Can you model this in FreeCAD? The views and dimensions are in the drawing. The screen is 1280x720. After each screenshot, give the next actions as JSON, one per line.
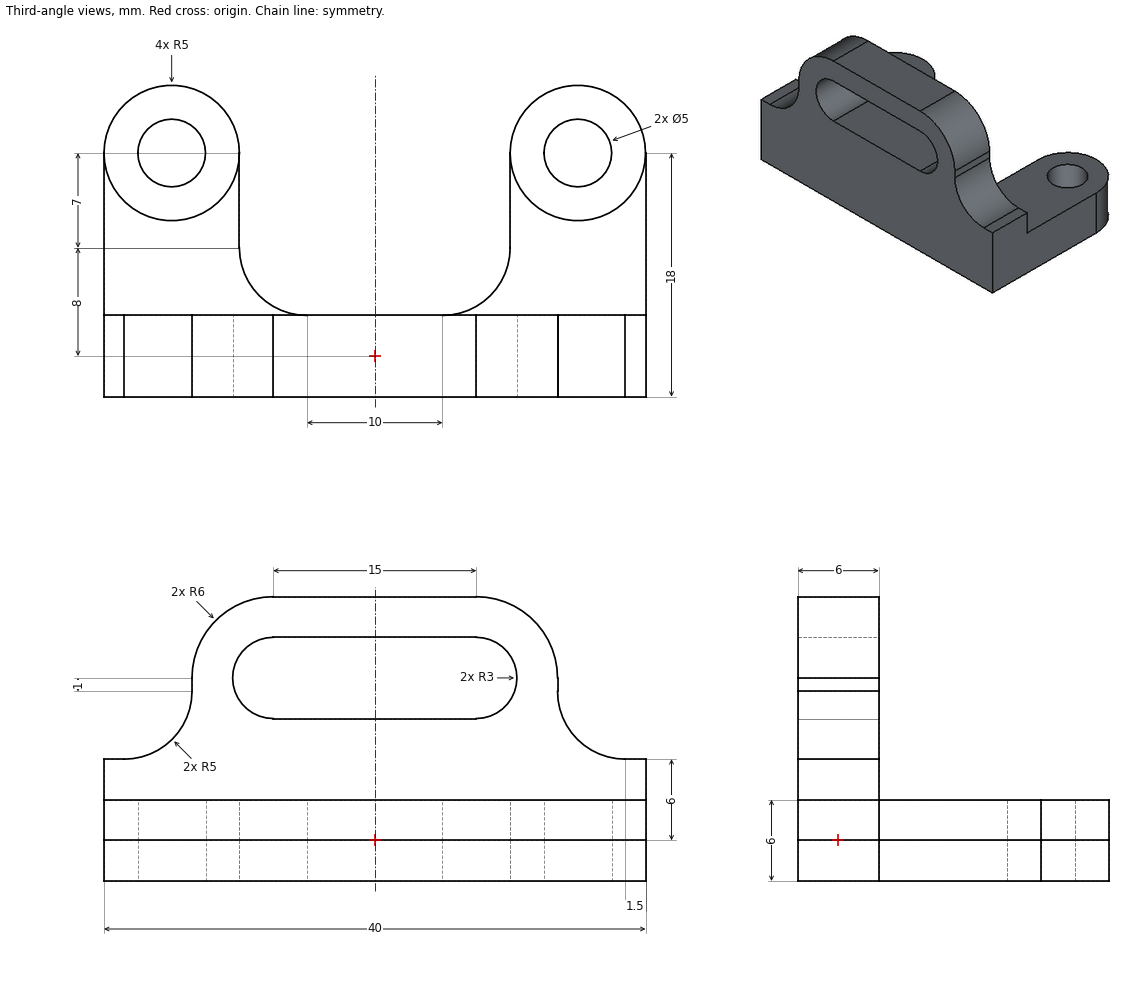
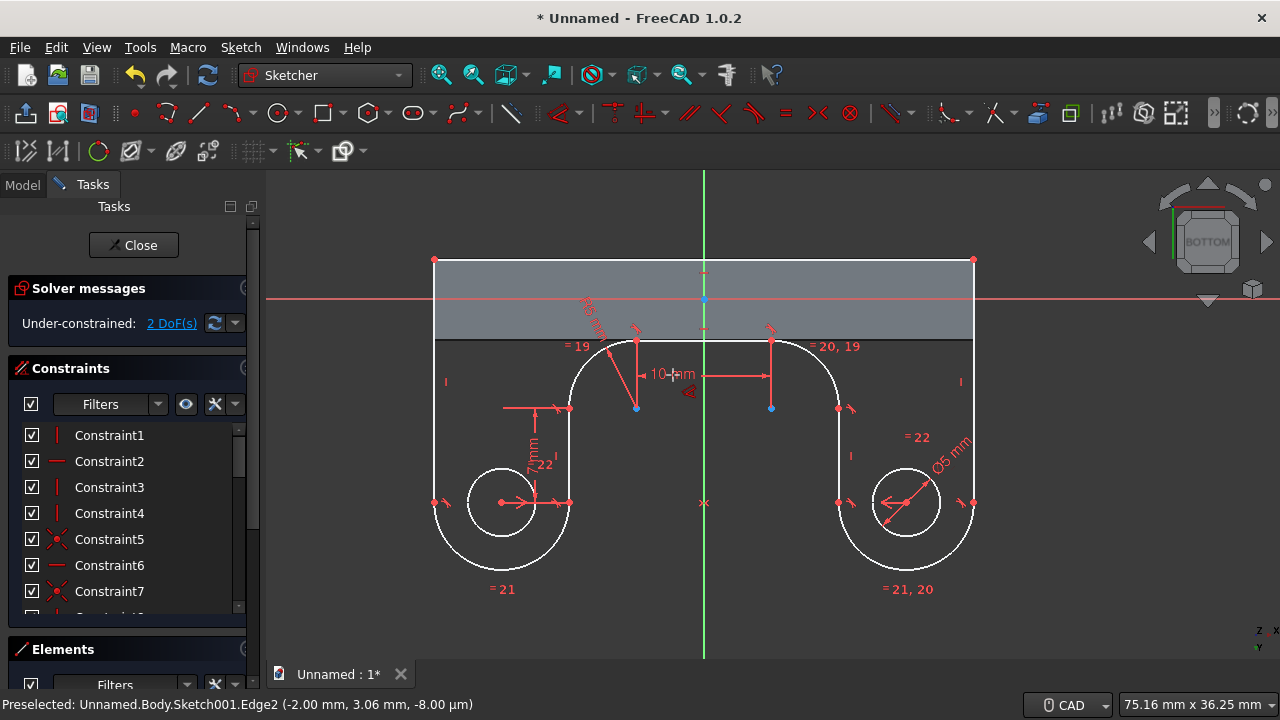
{"action": "left_click", "coordinate": [974, 430]}
{"action": "left_click", "coordinate": [1008, 381]}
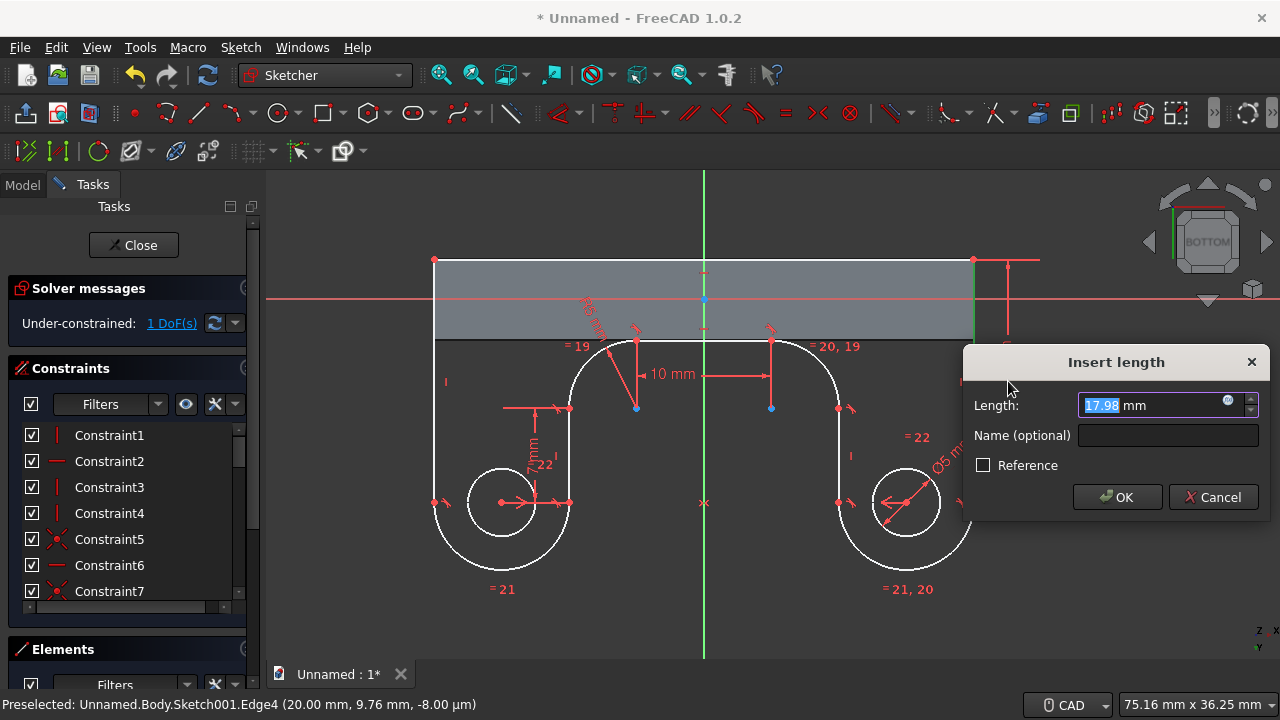
{"action": "type", "text": "18"}
{"action": "key", "text": "Return"}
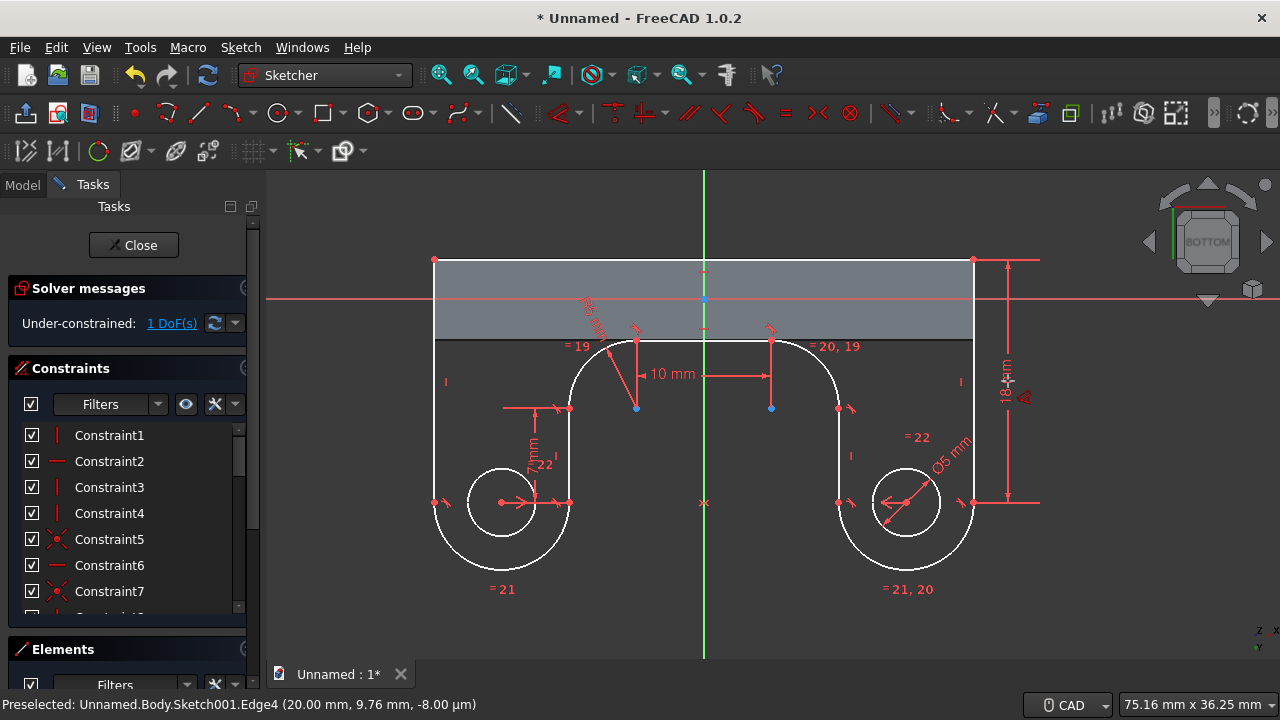
{"action": "left_click", "coordinate": [569, 408]}
{"action": "left_click", "coordinate": [535, 354]}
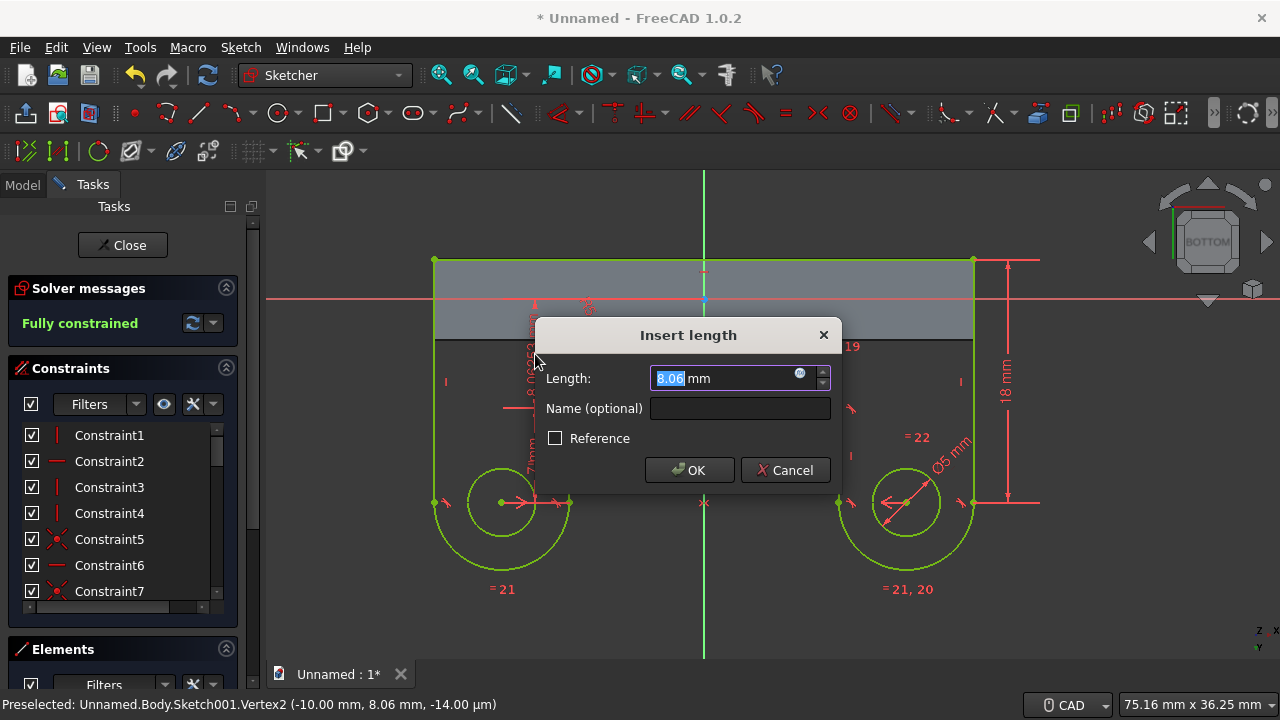
{"action": "type", "text": "8"}
{"action": "key", "text": "Return"}
{"action": "key", "text": "Escape"}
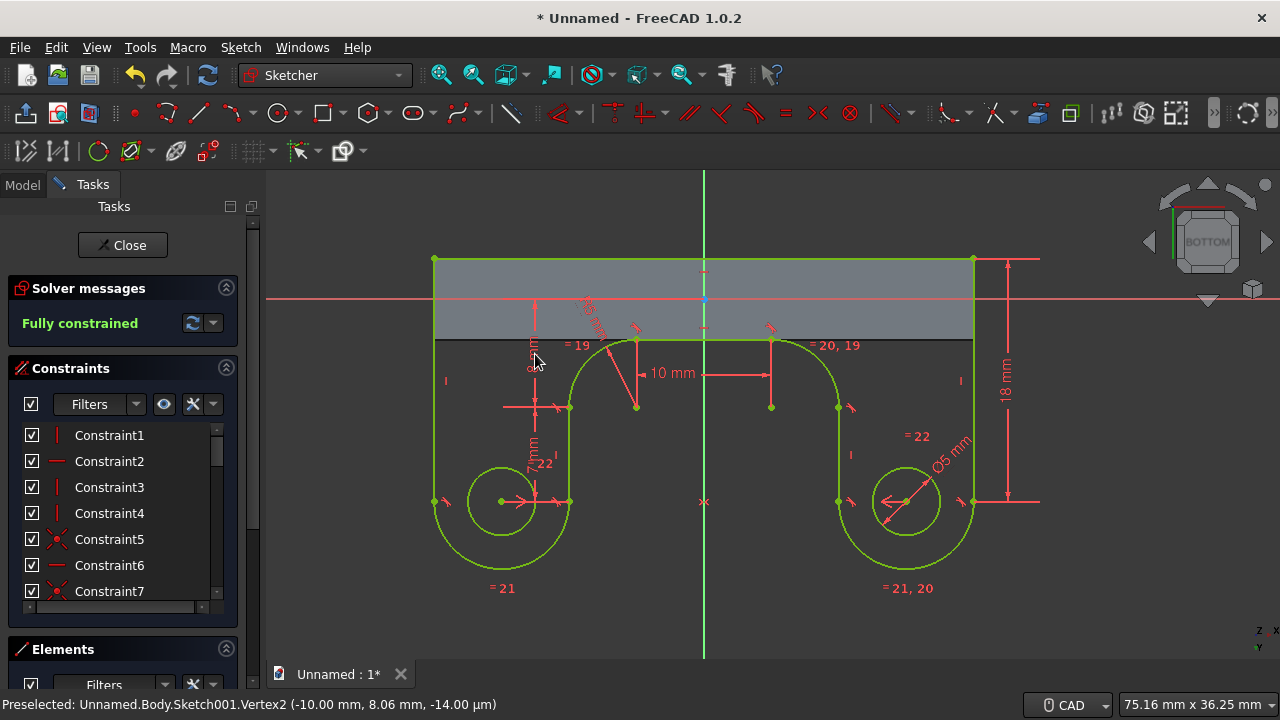
{"action": "left_click", "coordinate": [123, 245]}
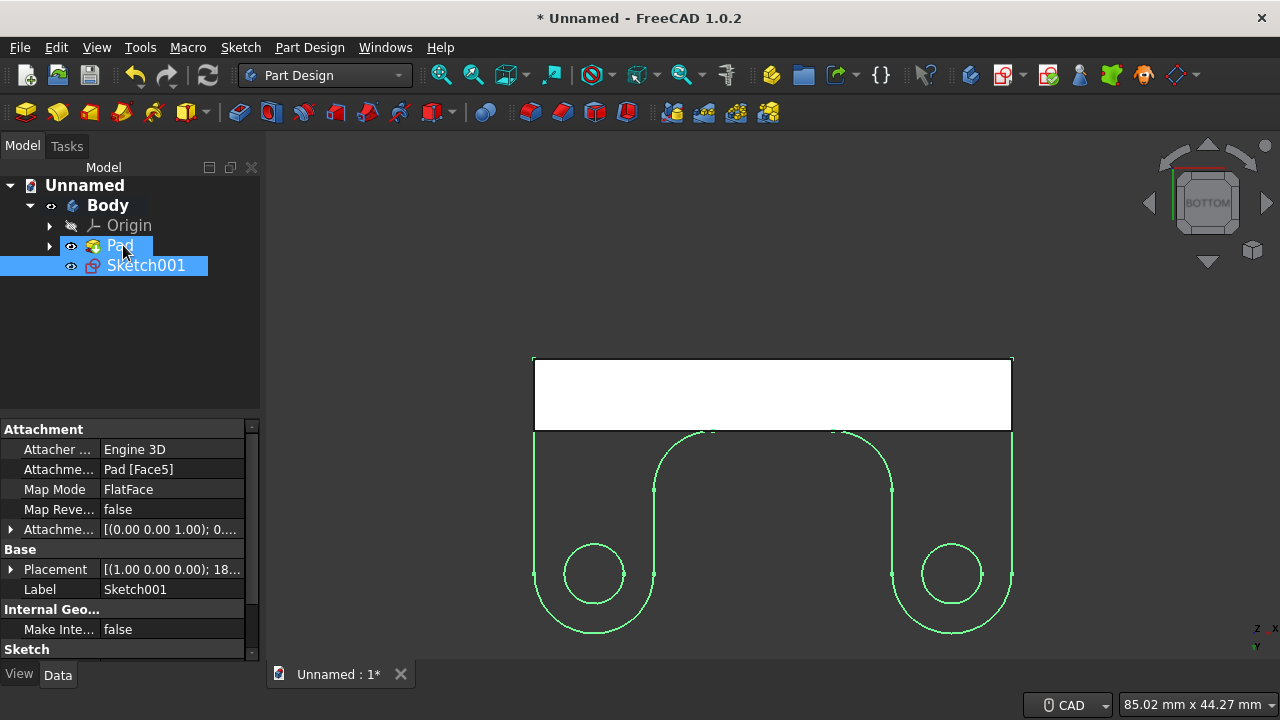
{"action": "left_click", "coordinate": [26, 112]}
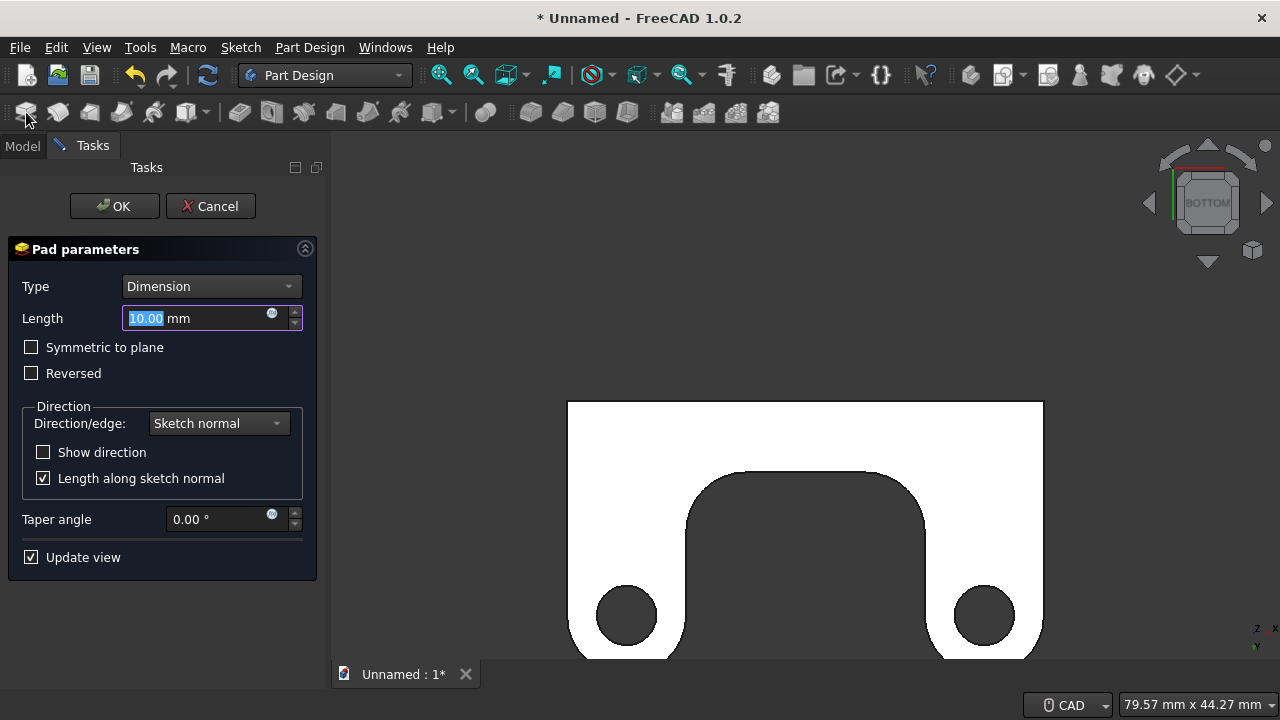
{"action": "type", "text": "6"}
{"action": "key", "text": "Tab"}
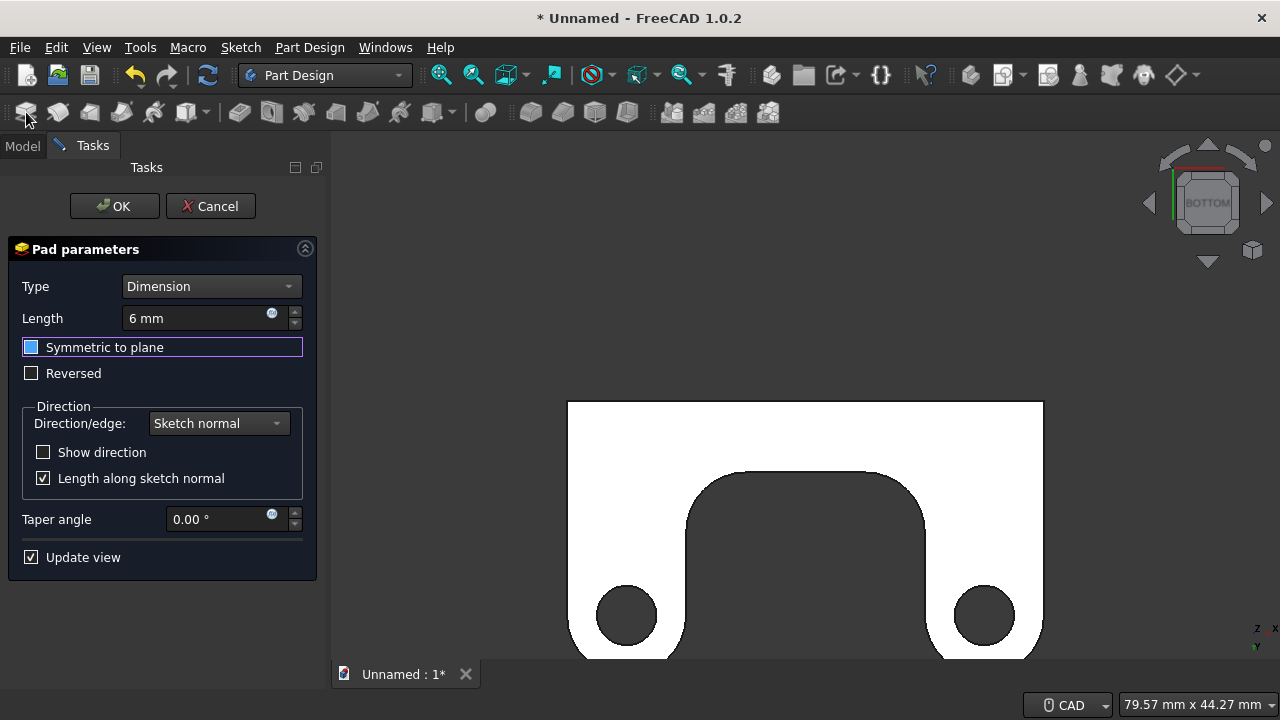
{"action": "left_click", "coordinate": [30, 347]}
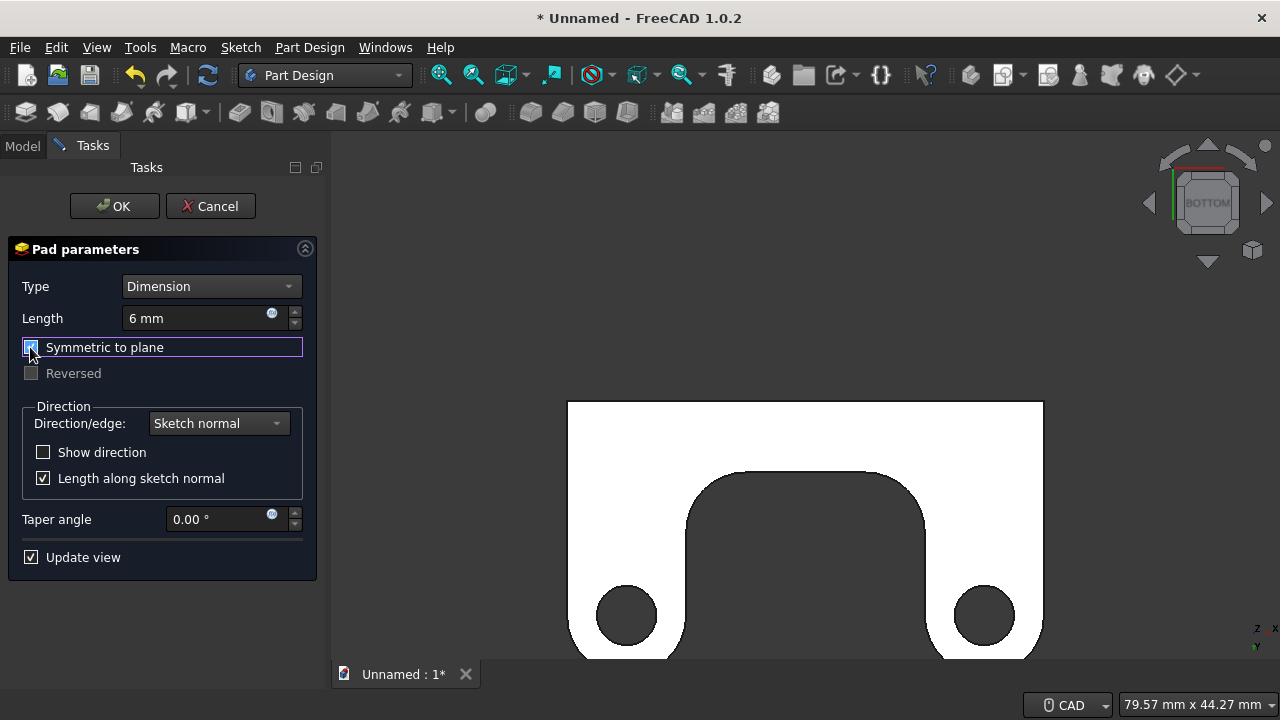
{"action": "left_click", "coordinate": [115, 206]}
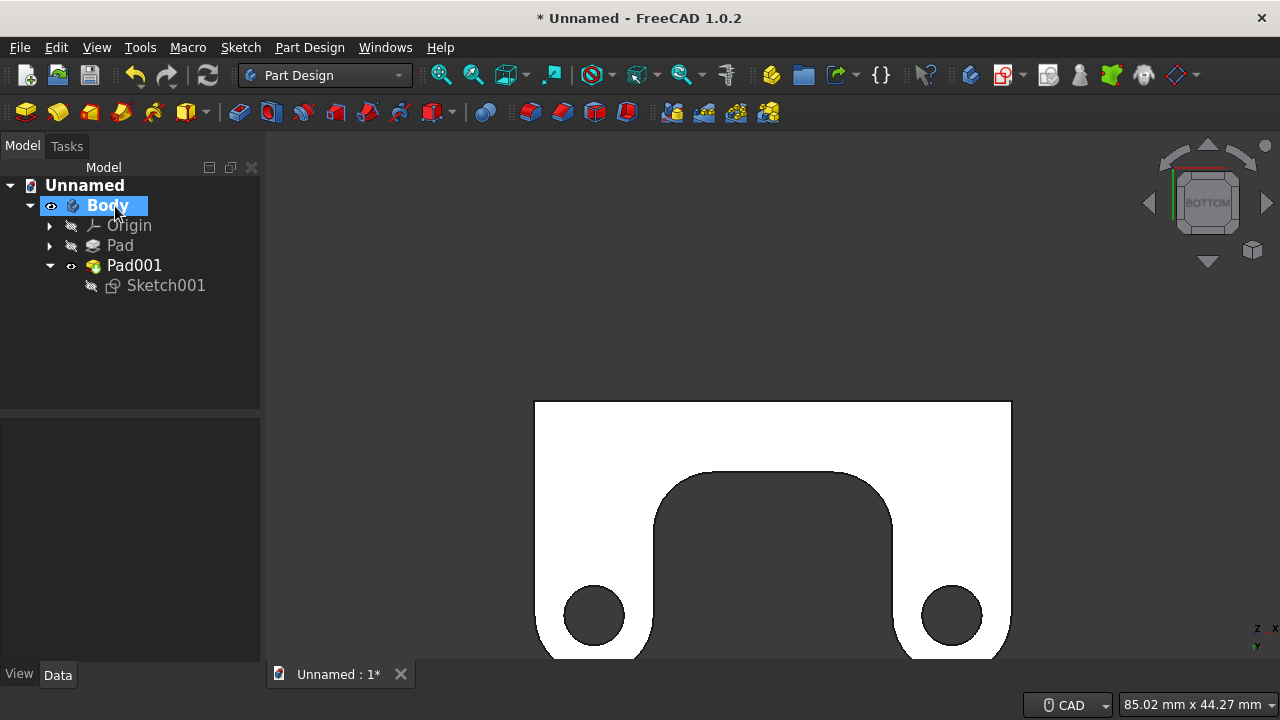
{"action": "key", "text": "0"}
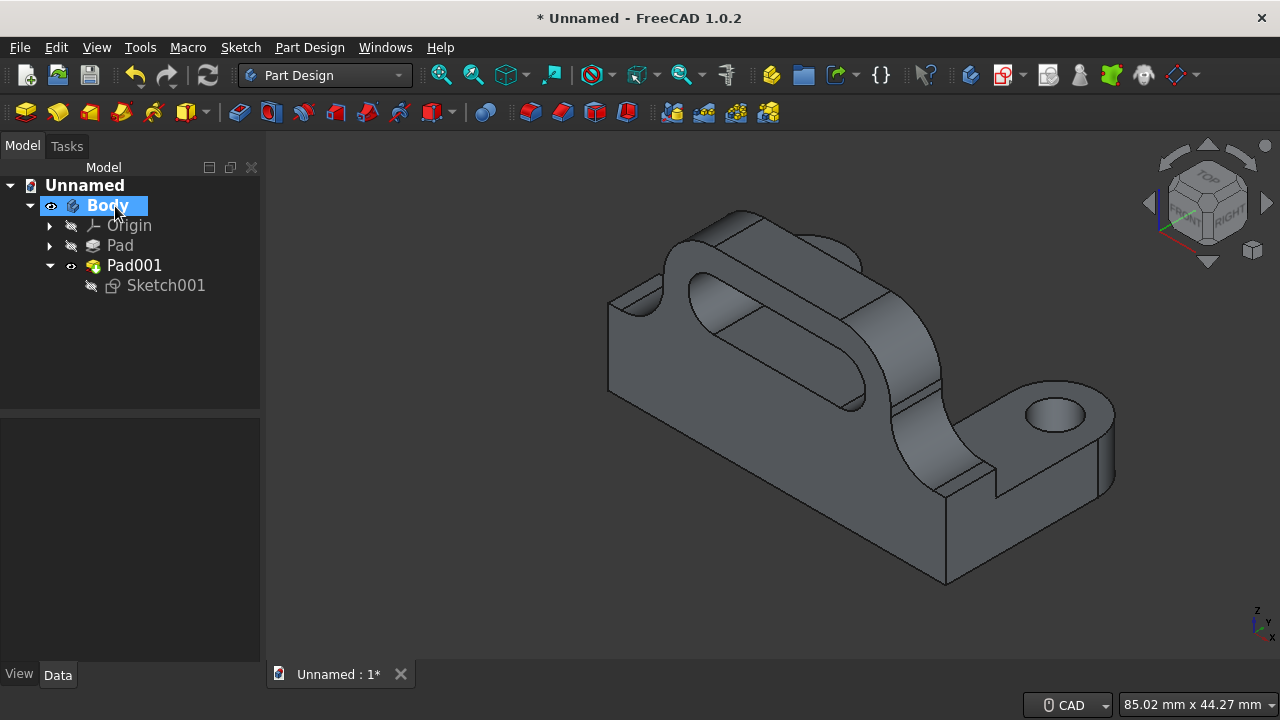
{"action": "left_click", "coordinate": [442, 76]}